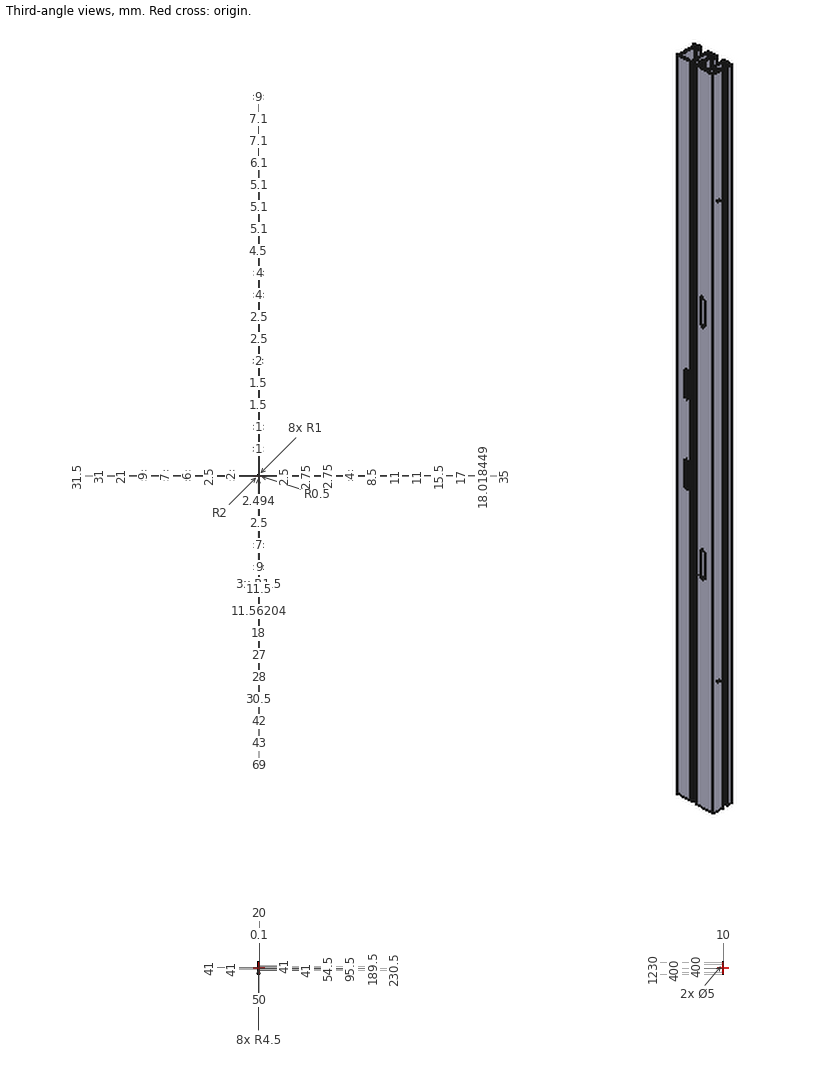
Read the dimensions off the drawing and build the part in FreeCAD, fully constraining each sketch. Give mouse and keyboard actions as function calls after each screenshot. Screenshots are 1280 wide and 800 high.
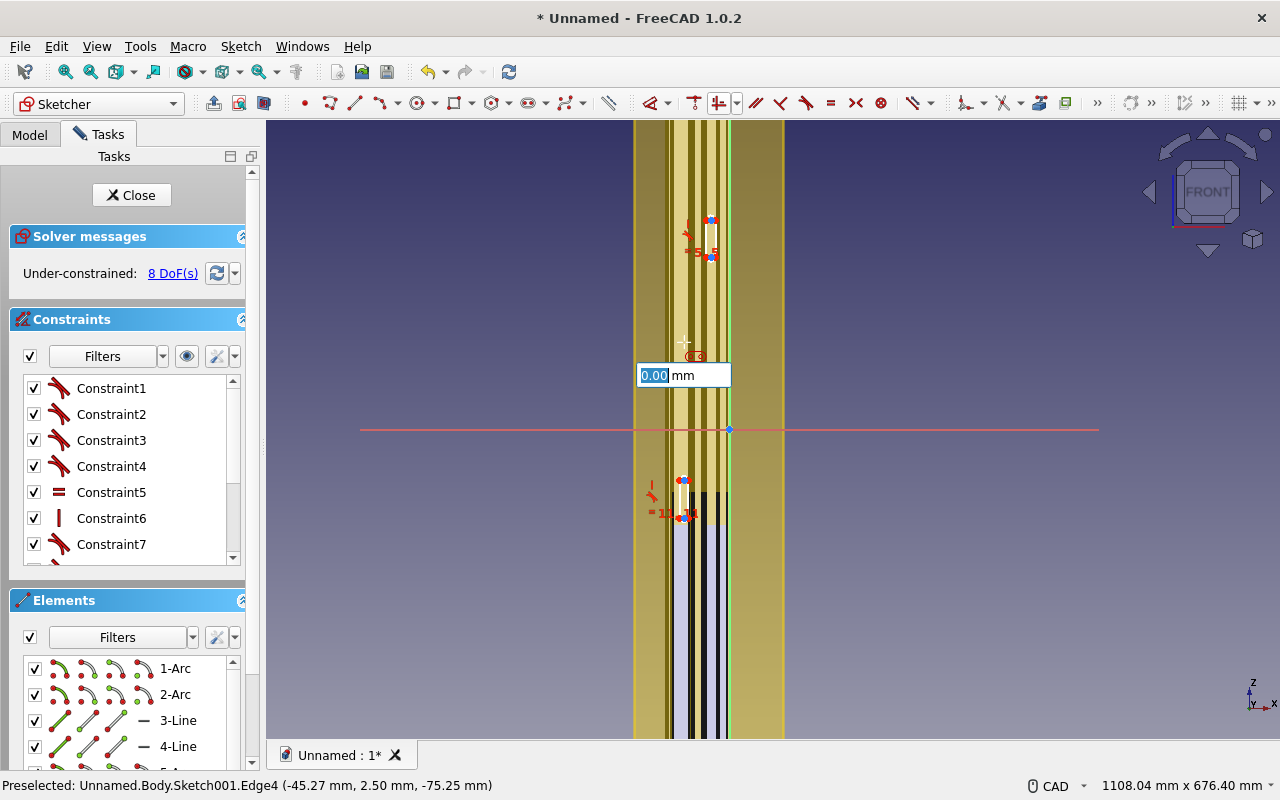
scroll(688, 361, up, 7)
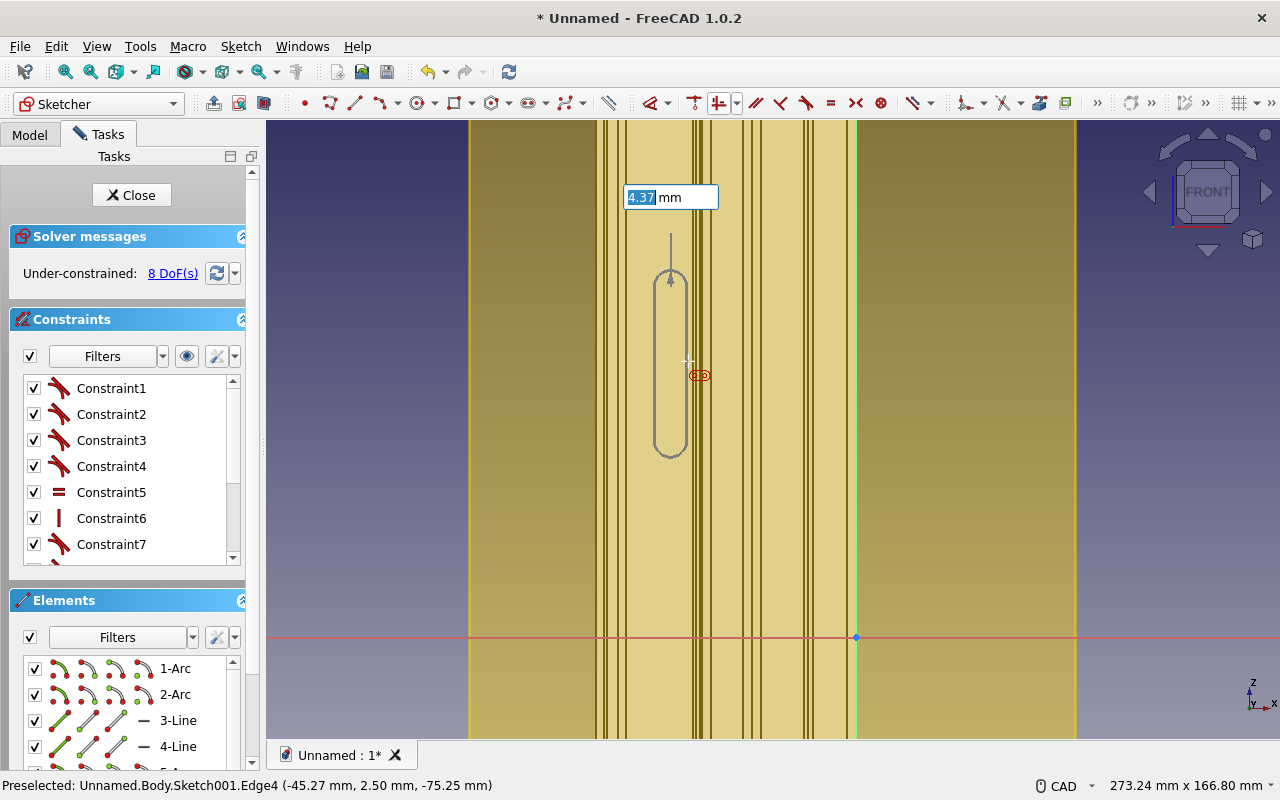
click(687, 360)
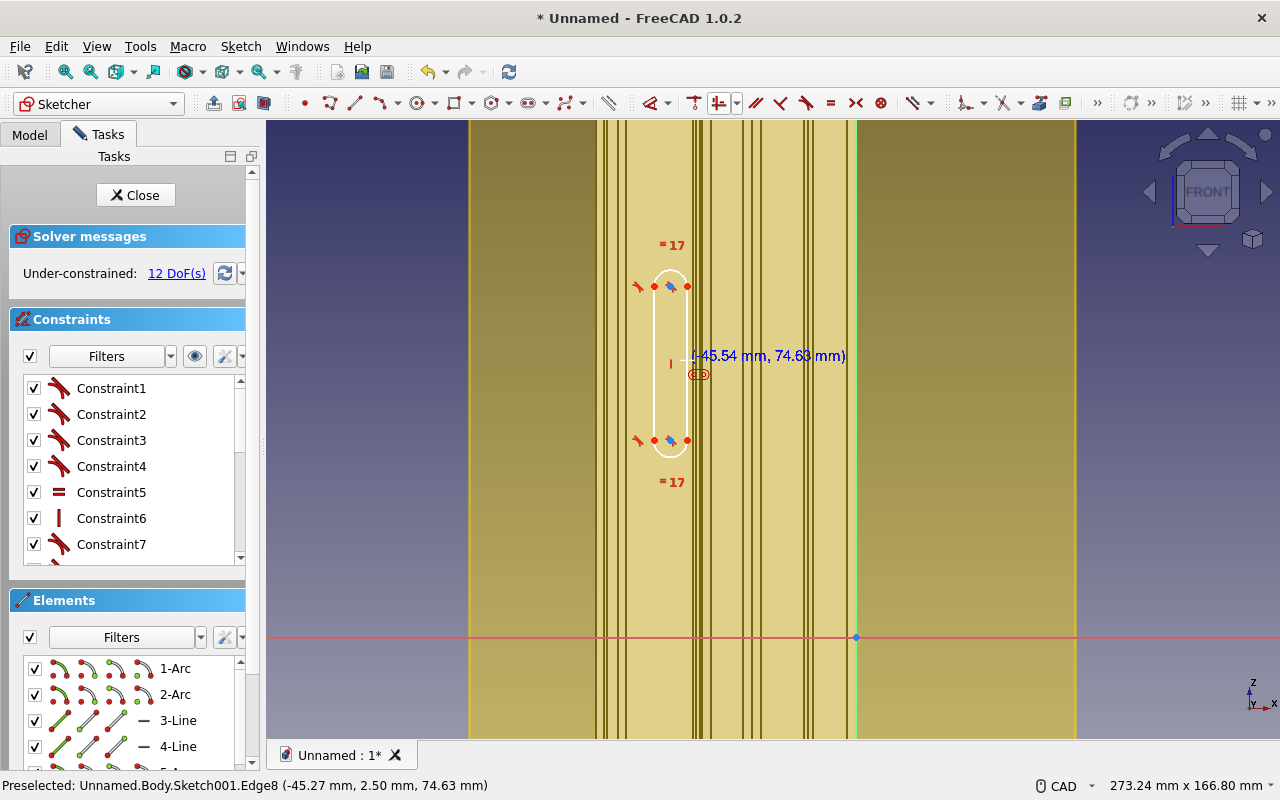
scroll(688, 361, down, 7)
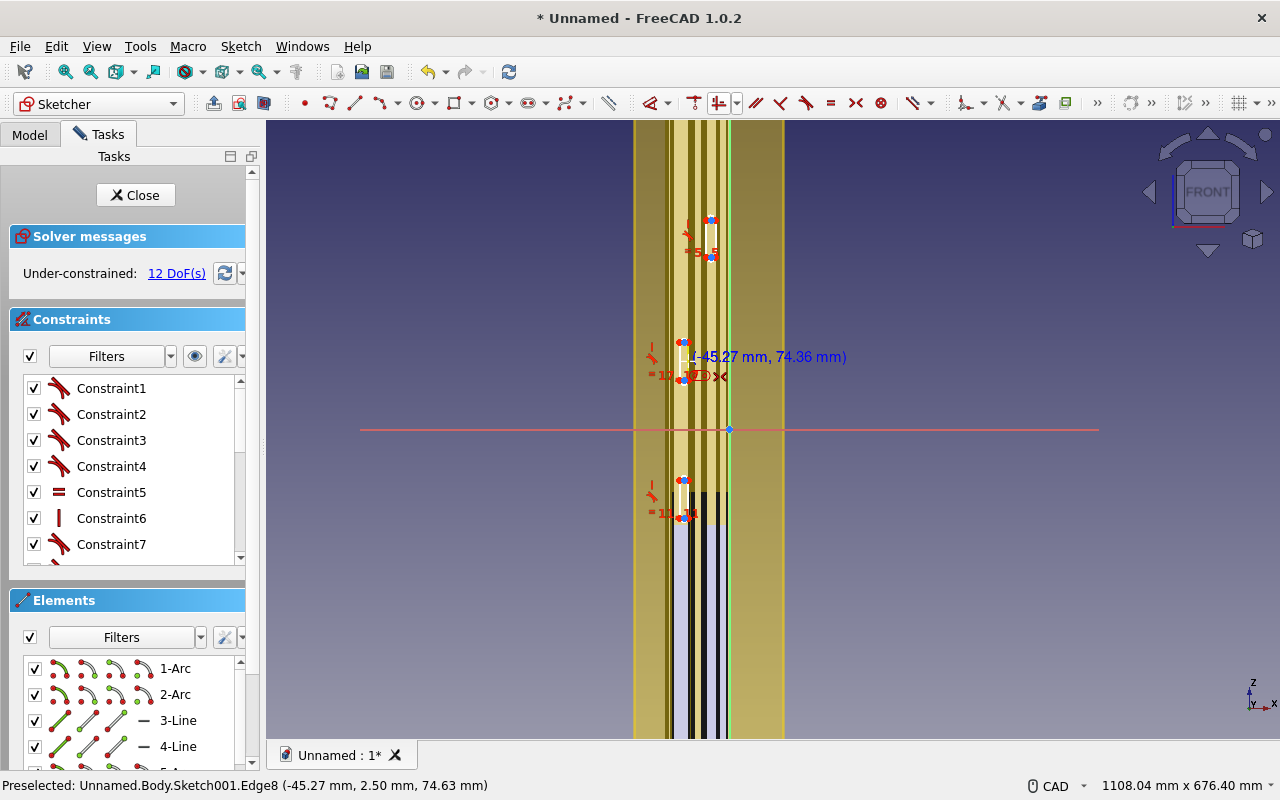
scroll(711, 641, up, 9)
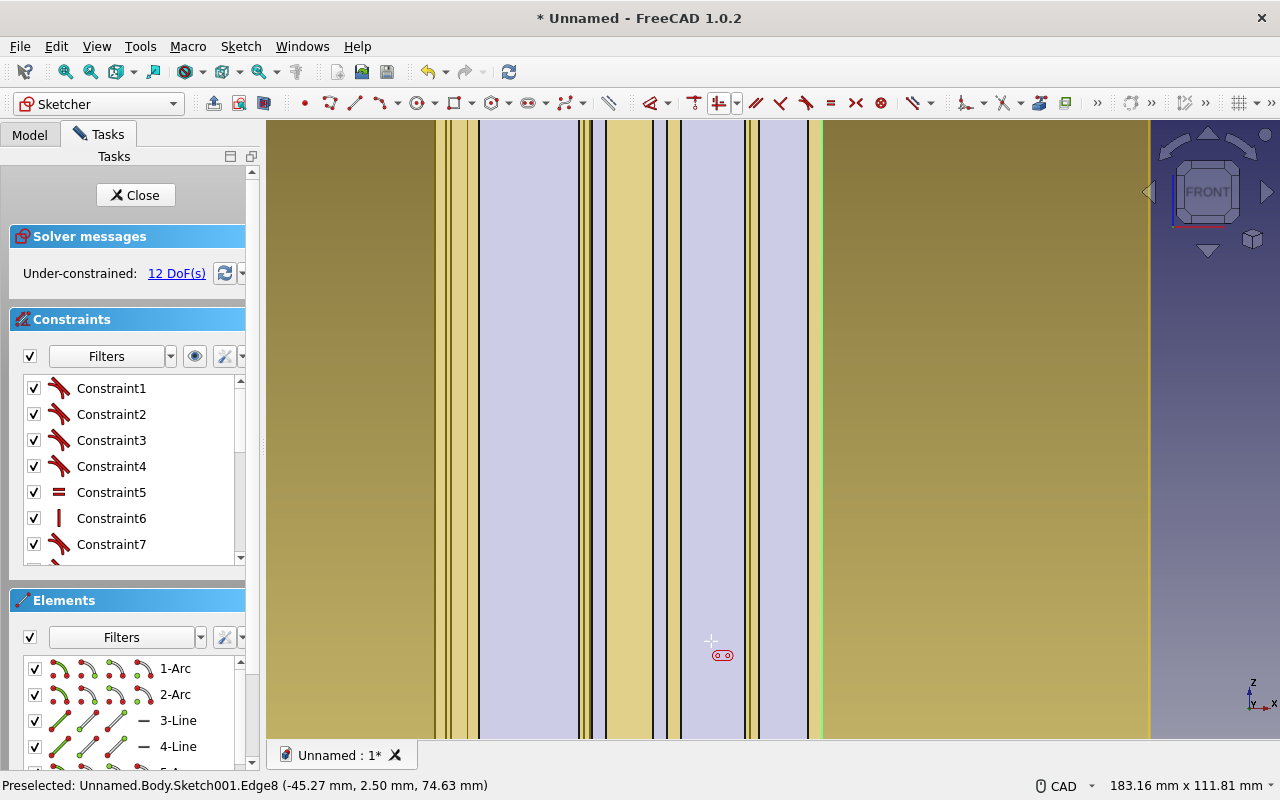
scroll(711, 642, down, 9)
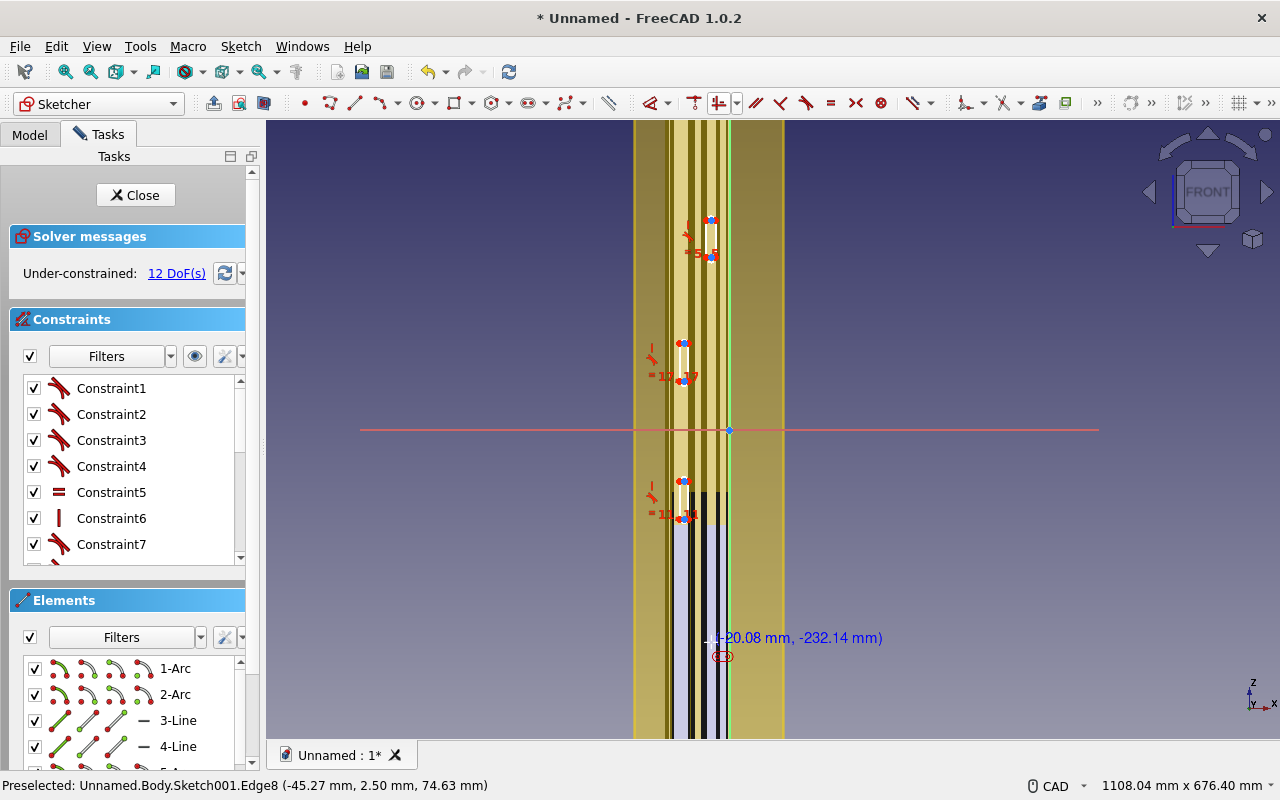
click(711, 641)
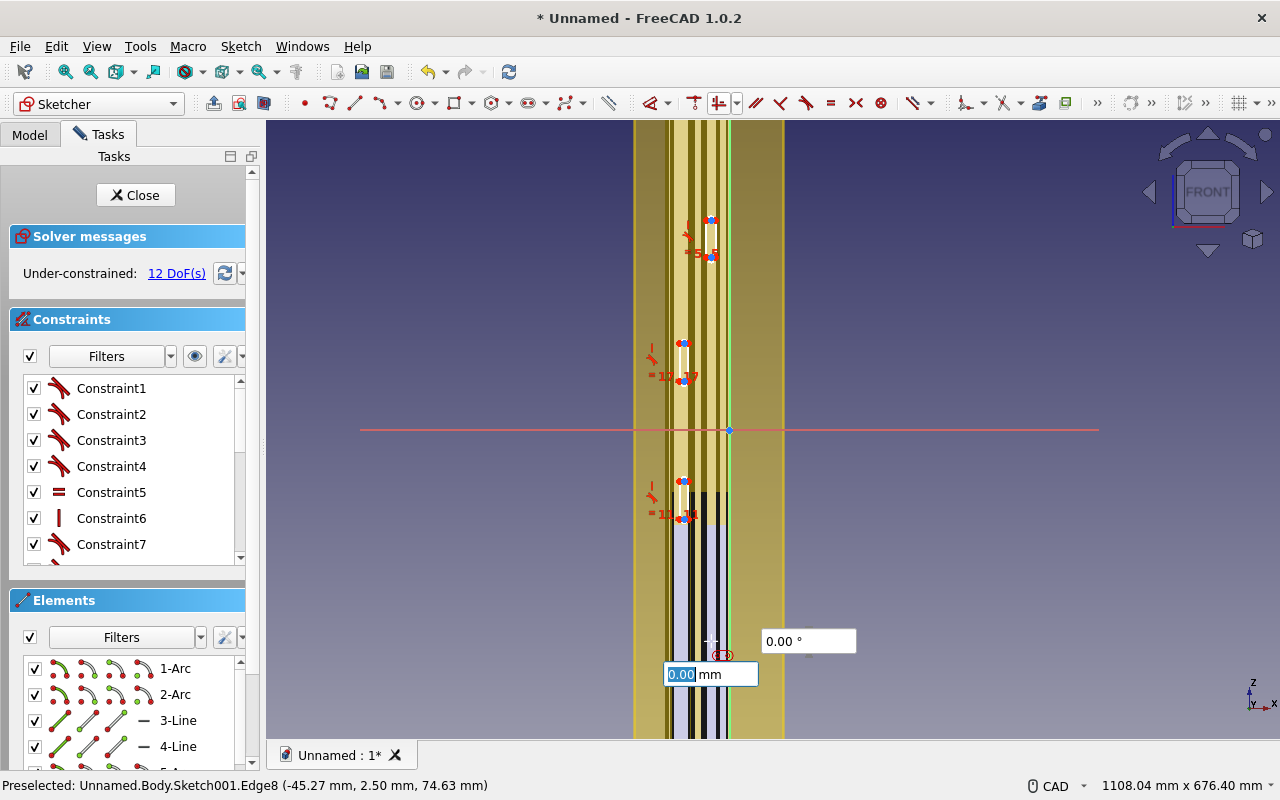
click(711, 604)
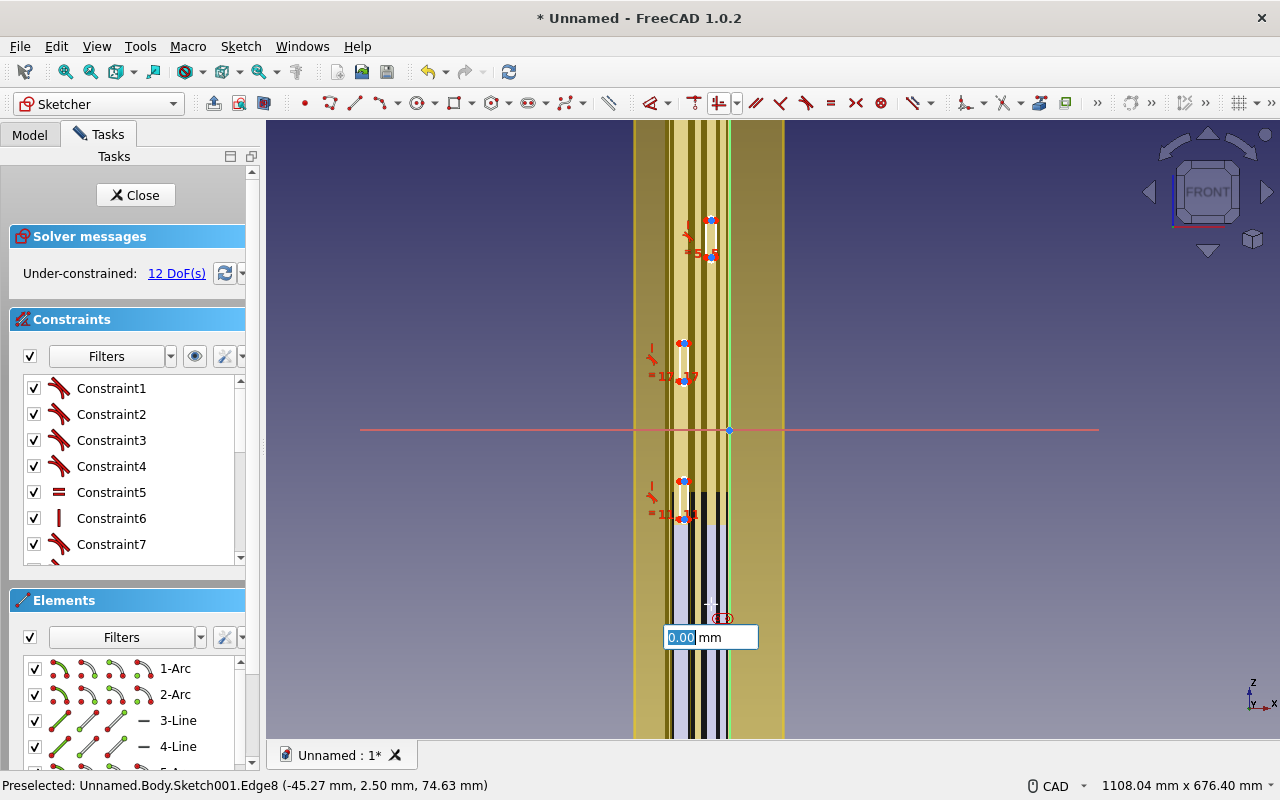
scroll(716, 623, up, 7)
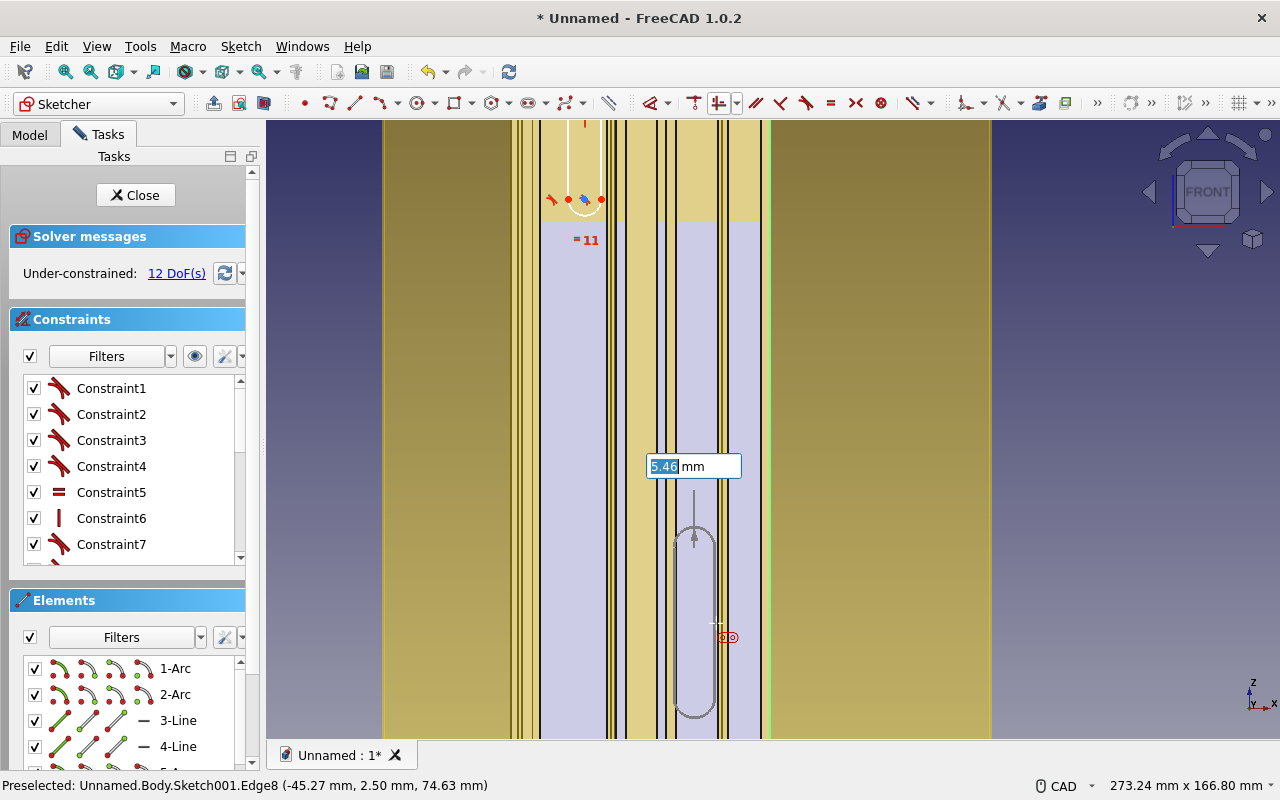
click(713, 619)
key(Escape)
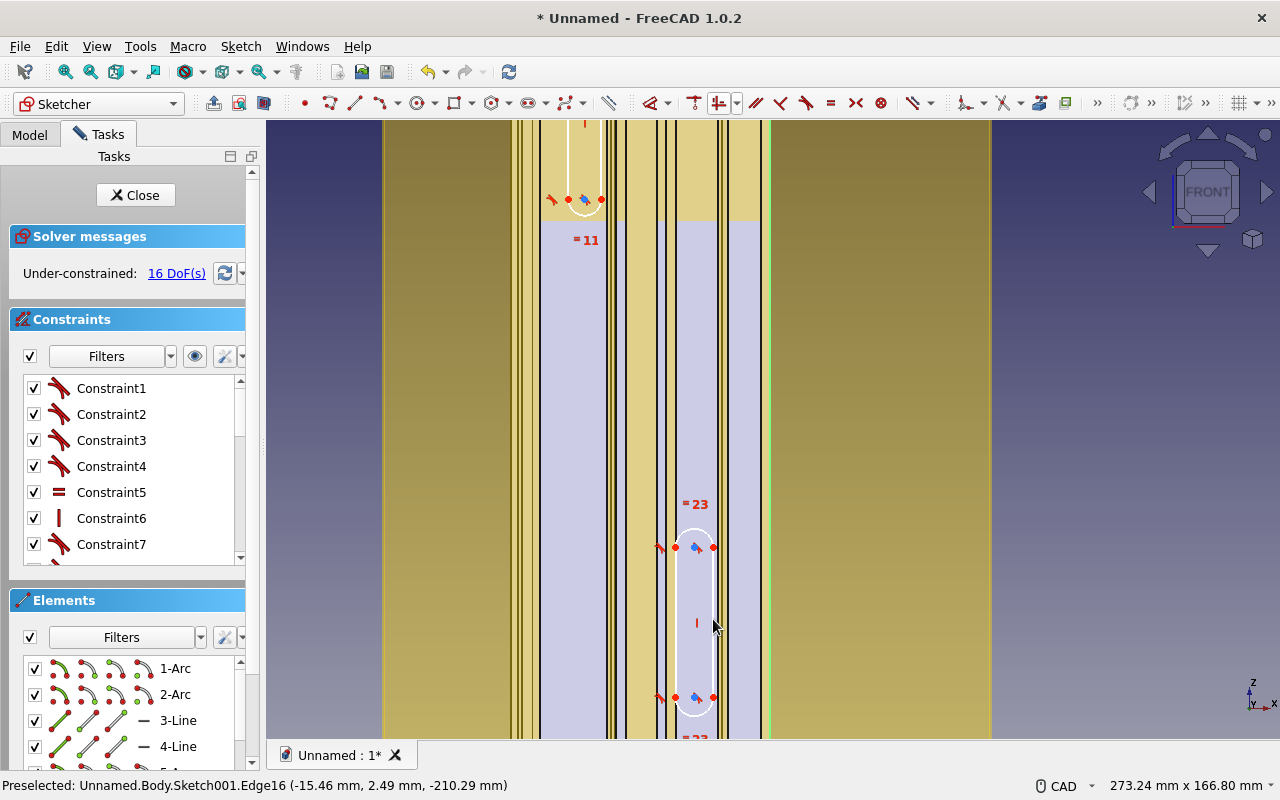
scroll(716, 623, down, 7)